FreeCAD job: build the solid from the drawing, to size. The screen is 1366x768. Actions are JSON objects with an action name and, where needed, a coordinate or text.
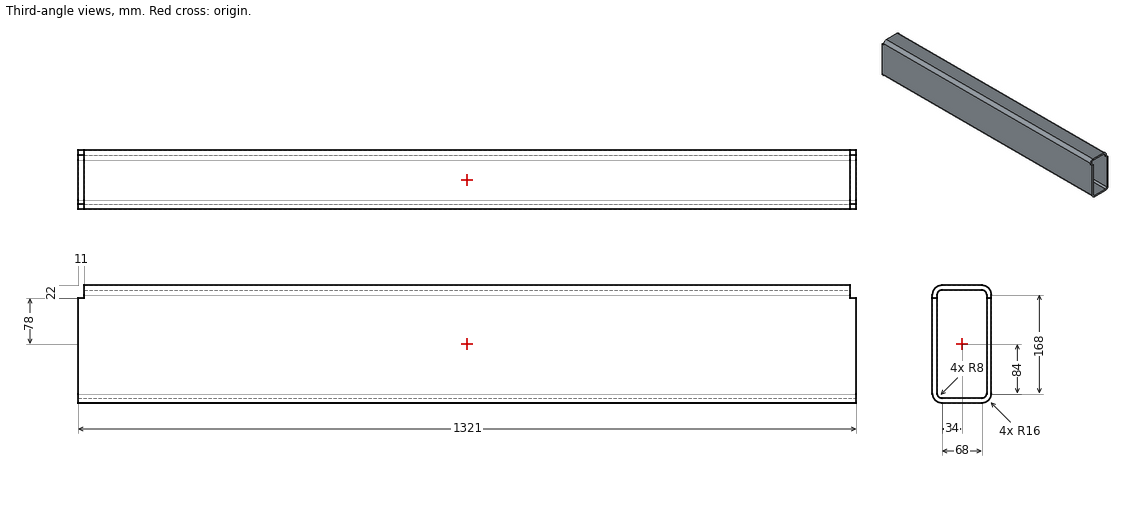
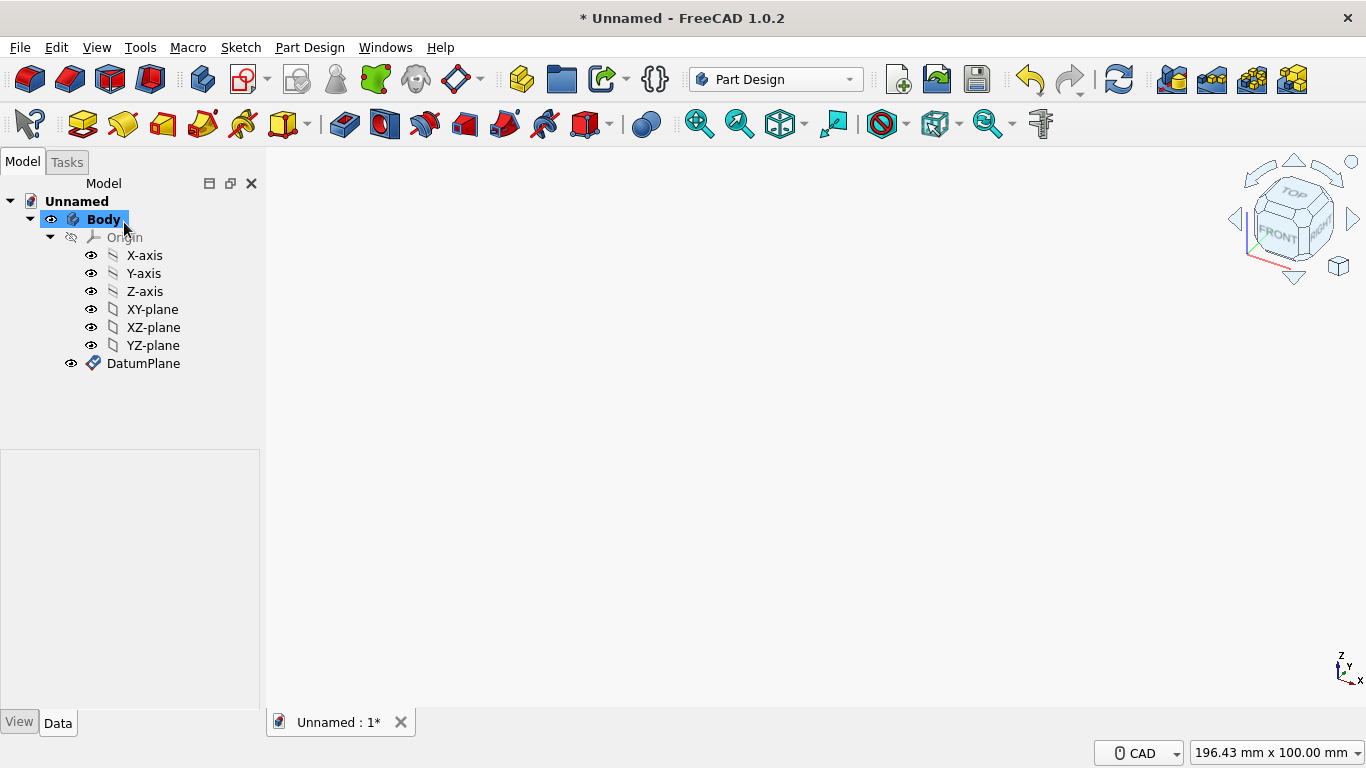
{"action": "left_click", "coordinate": [116, 363]}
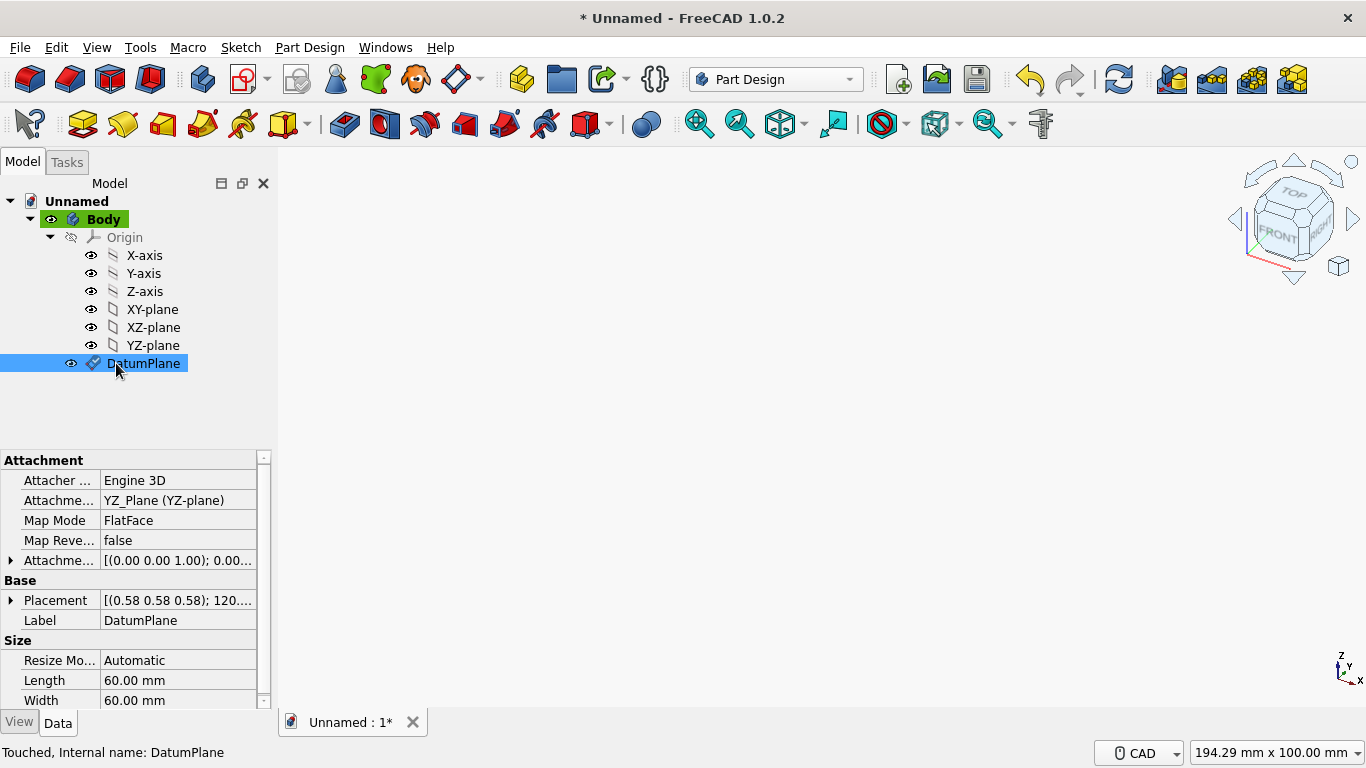
{"action": "left_click", "coordinate": [244, 80]}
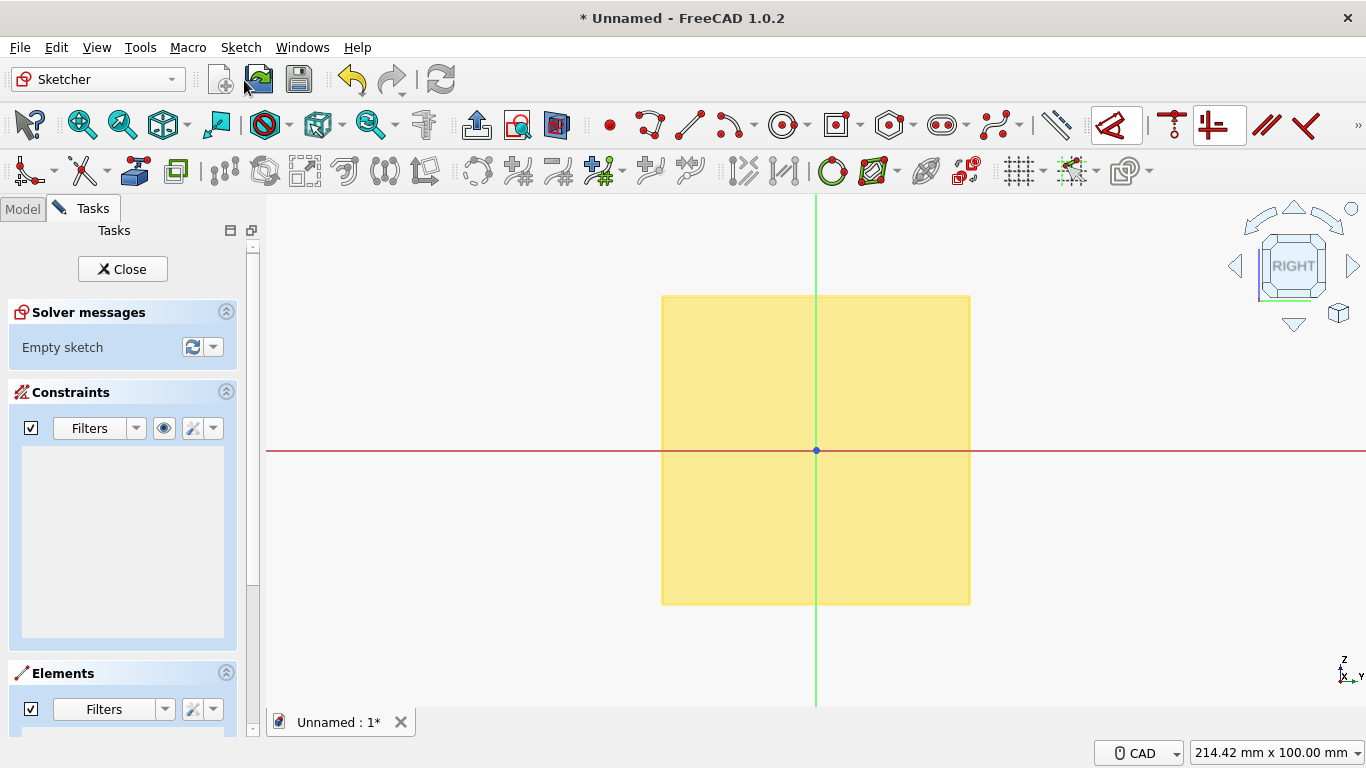
{"action": "scroll", "coordinate": [718, 450], "scroll_direction": "down", "scroll_amount": 6}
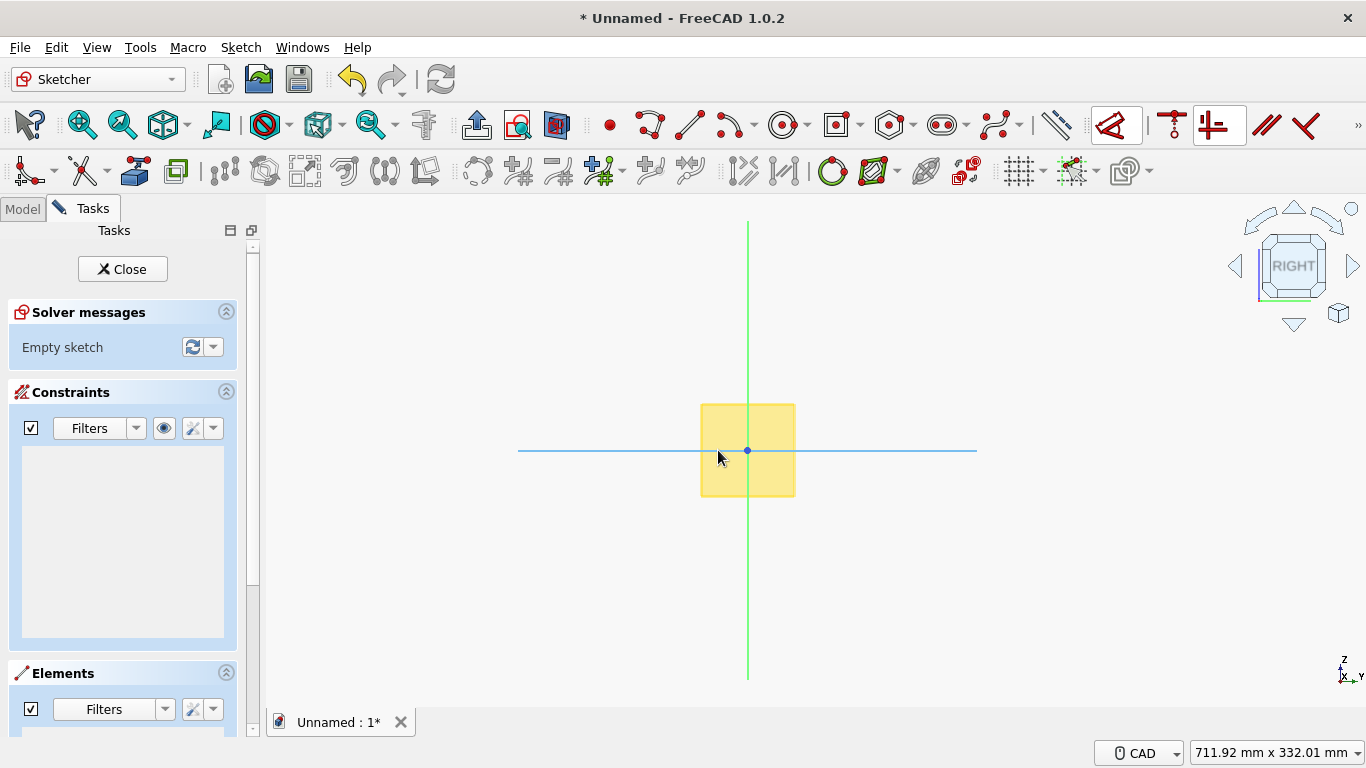
{"action": "key", "text": "g l"}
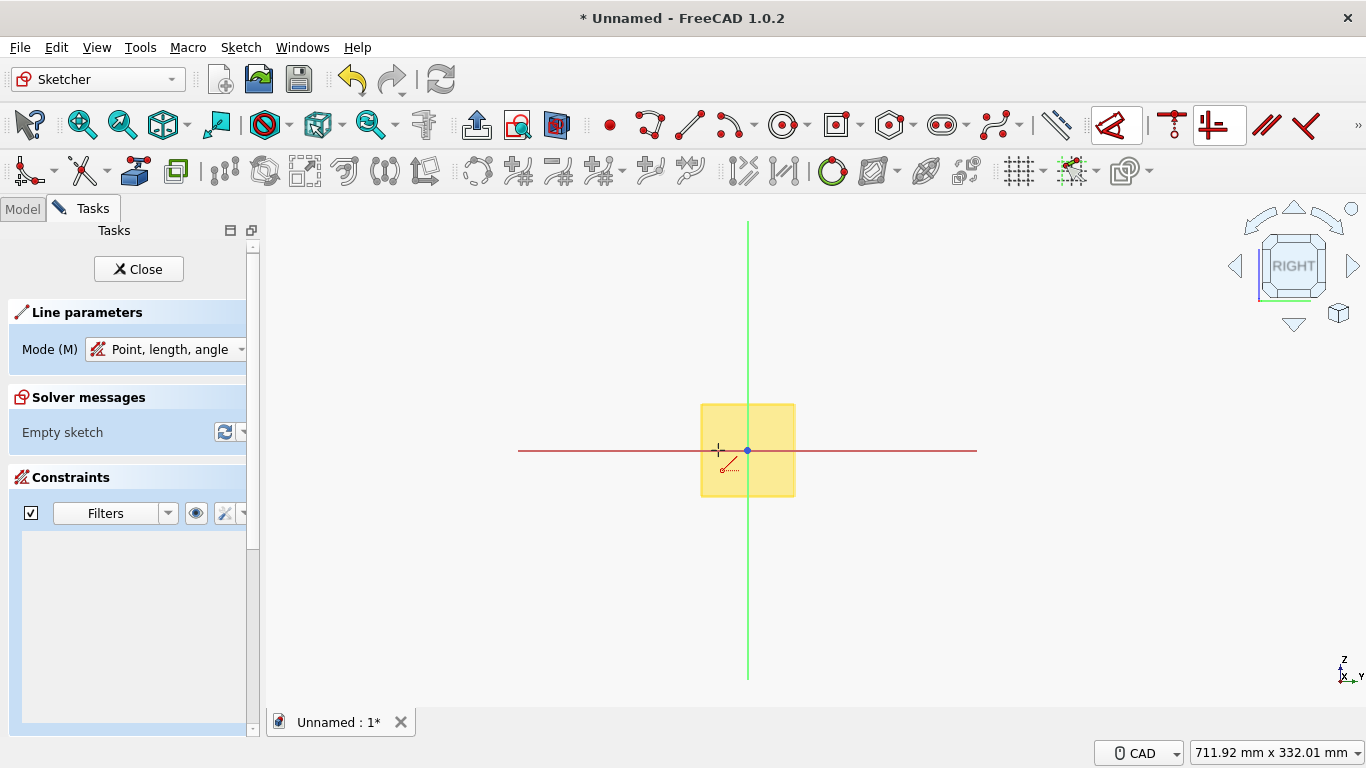
{"action": "left_click", "coordinate": [695, 605]}
{"action": "left_click", "coordinate": [800, 605]}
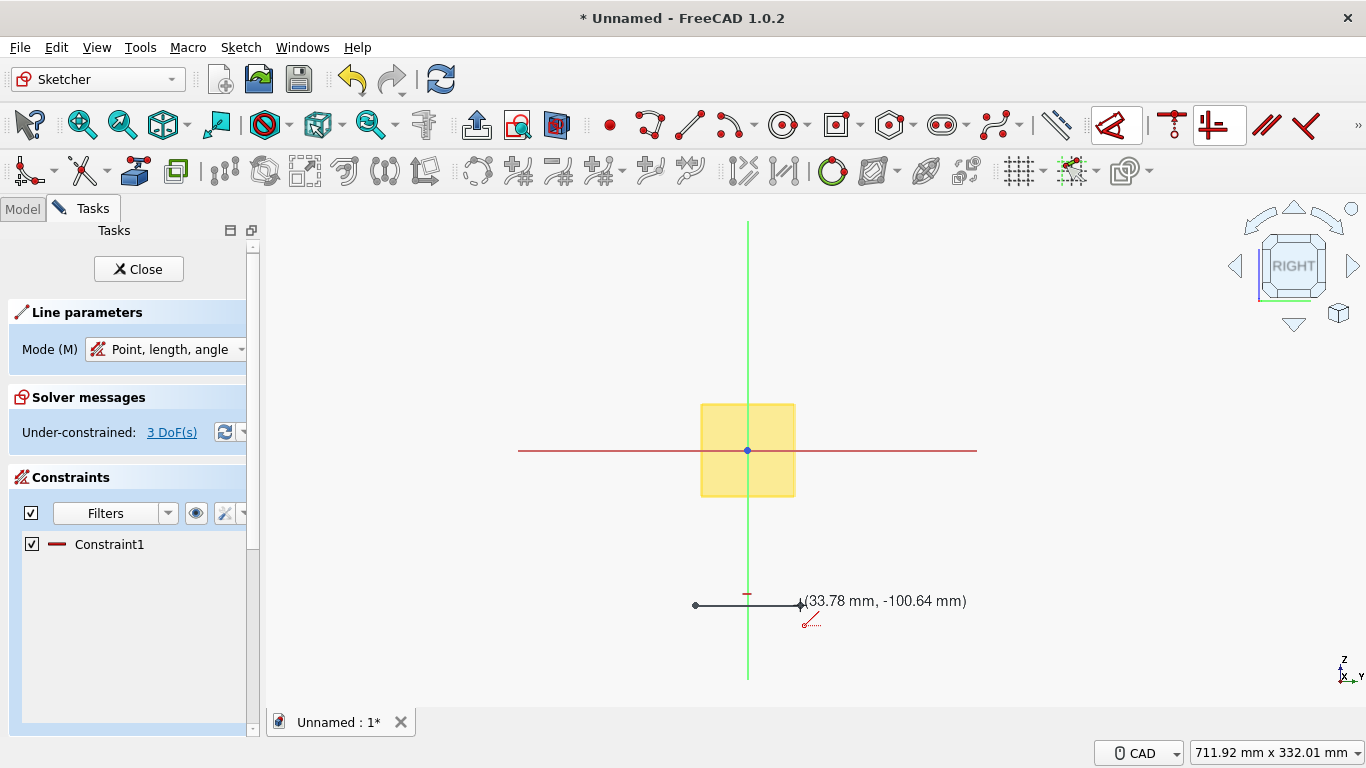
{"action": "left_click", "coordinate": [825, 580]}
{"action": "left_click", "coordinate": [825, 321]}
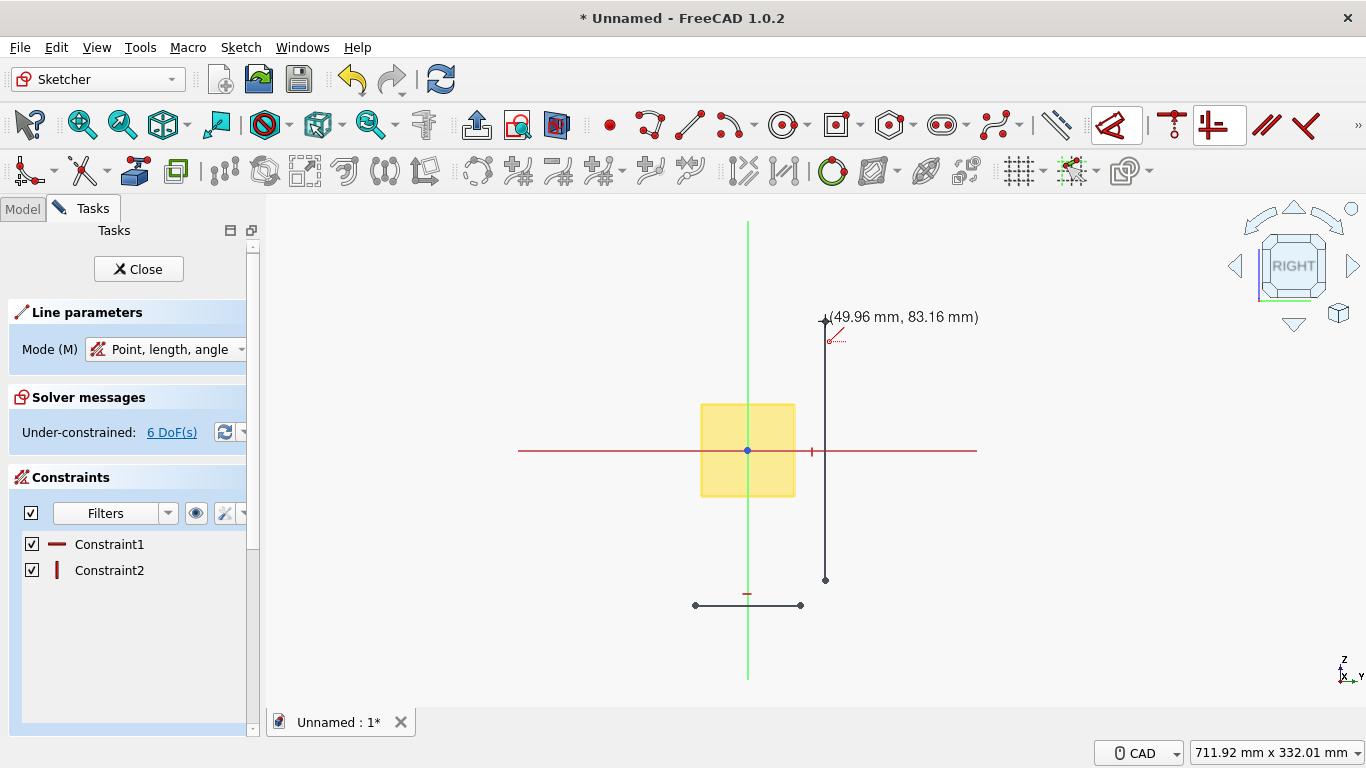
{"action": "left_click", "coordinate": [800, 296]}
{"action": "left_click", "coordinate": [695, 296]}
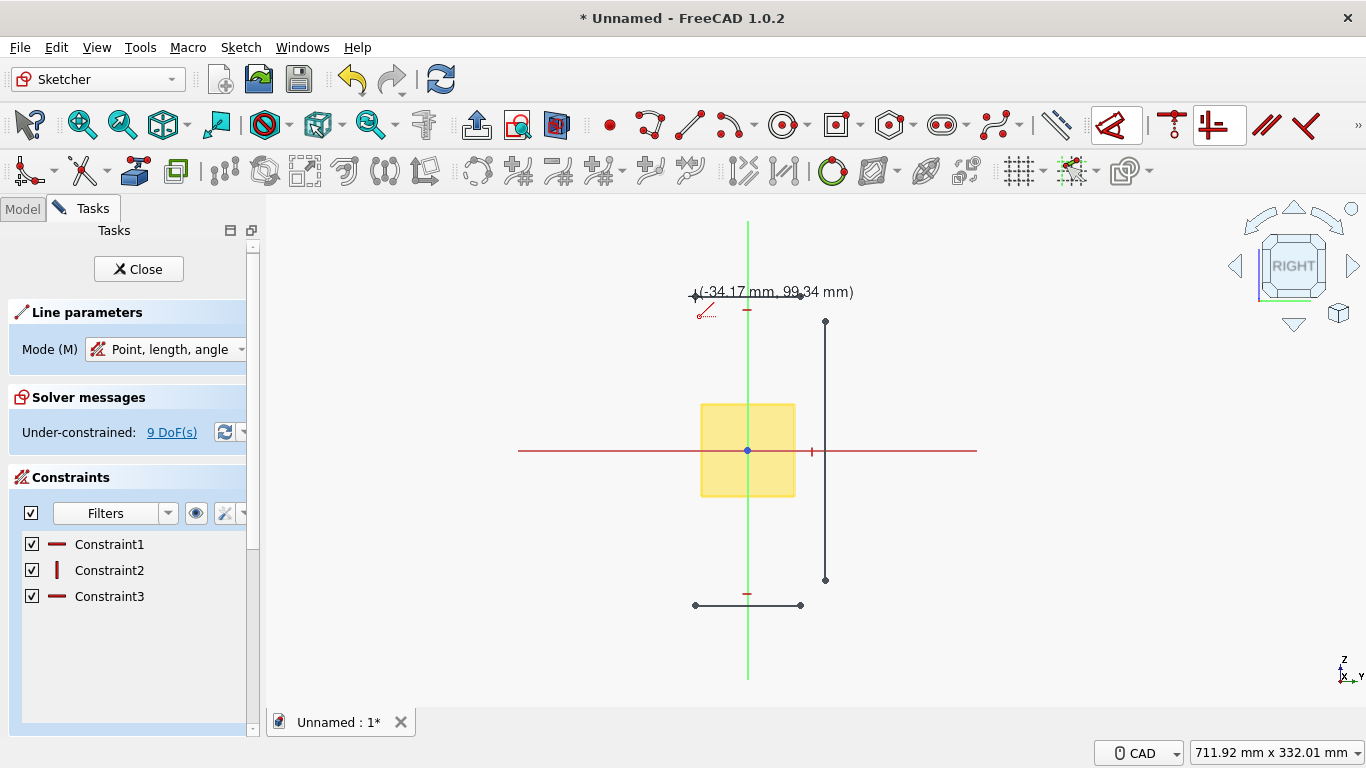
{"action": "left_click", "coordinate": [671, 321]}
{"action": "left_click", "coordinate": [671, 580]}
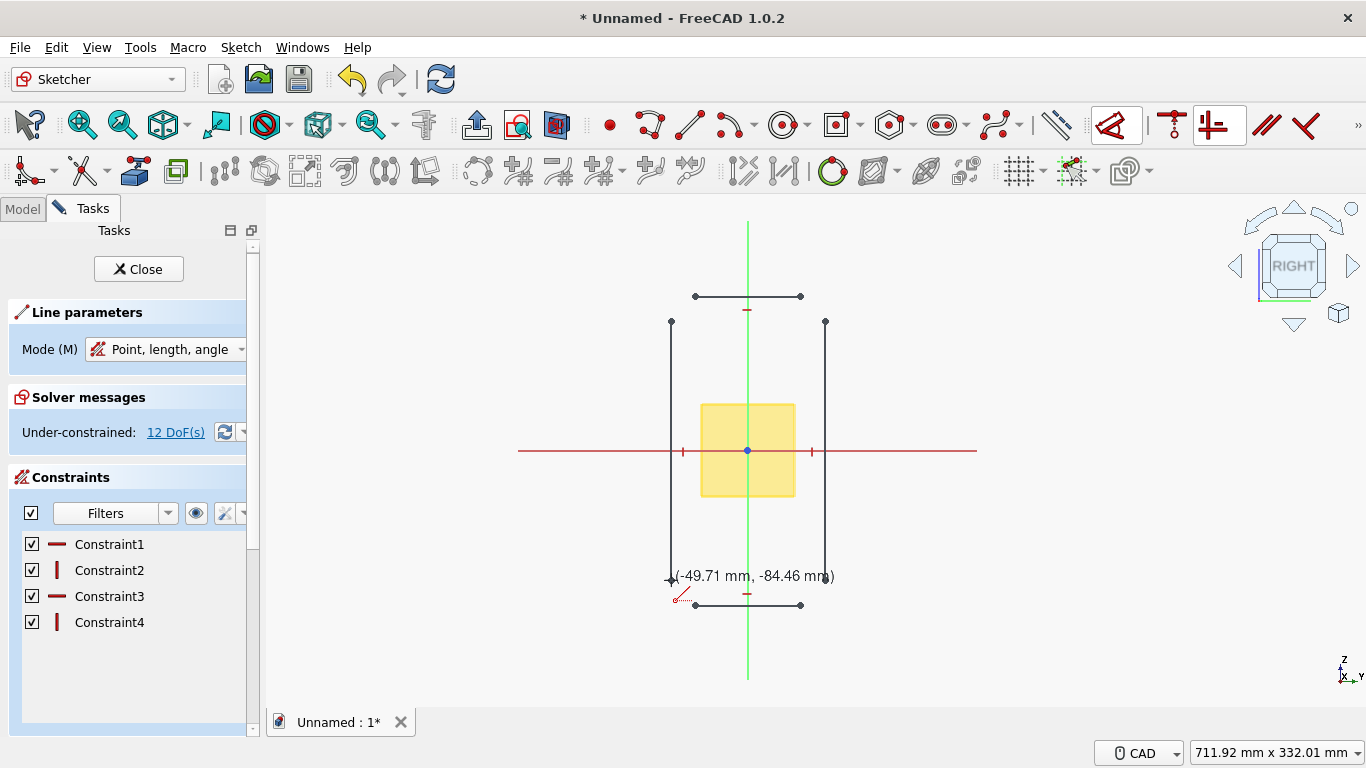
{"action": "key", "text": "g 3 a"}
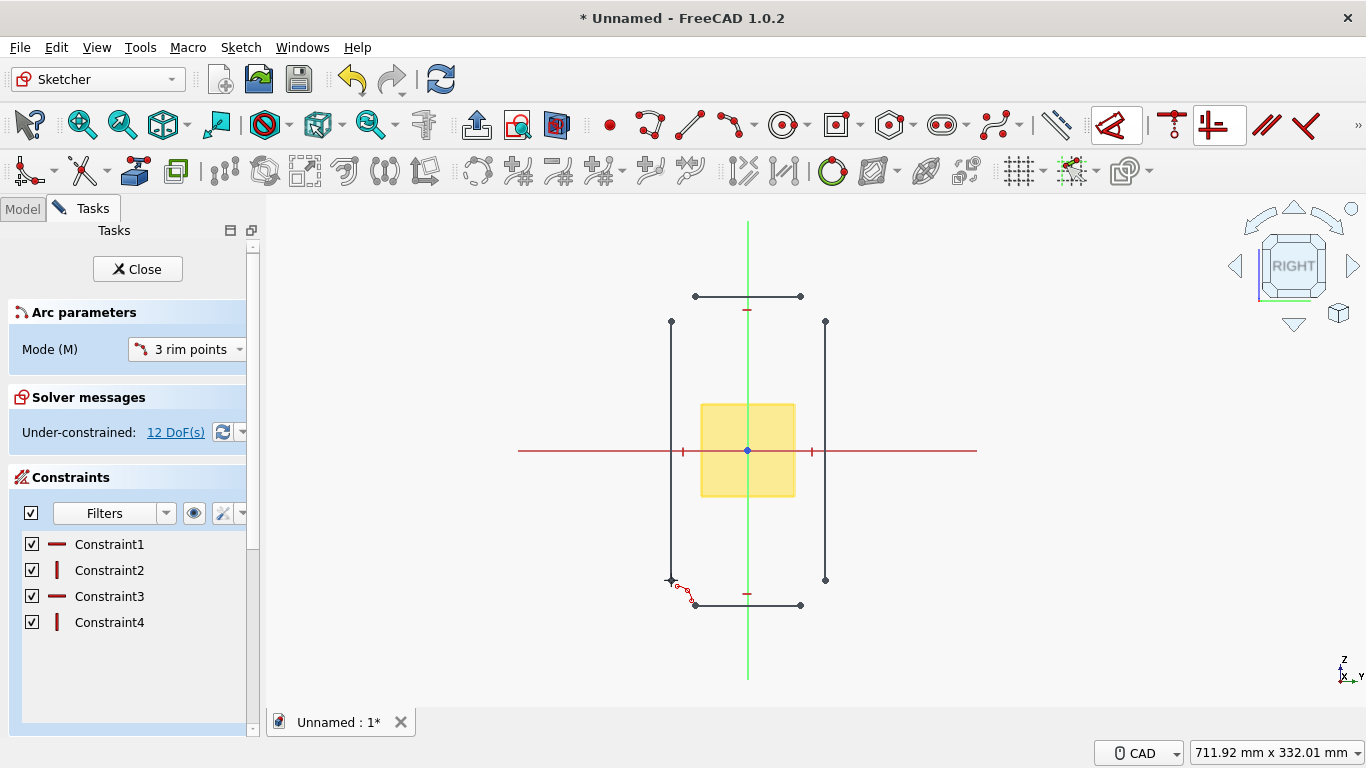
{"action": "left_click", "coordinate": [800, 606]}
{"action": "left_click", "coordinate": [825, 581]}